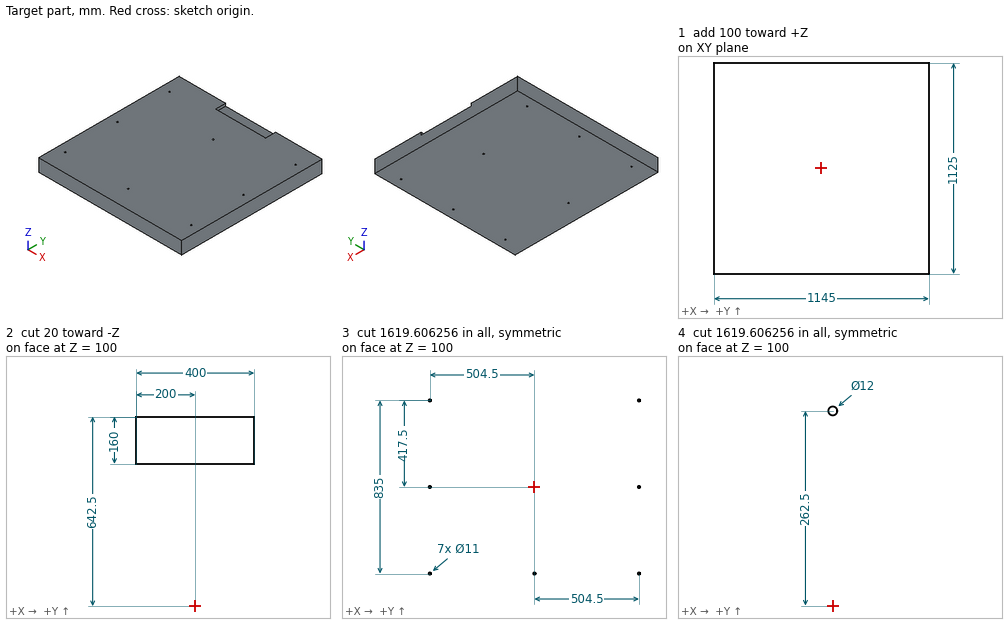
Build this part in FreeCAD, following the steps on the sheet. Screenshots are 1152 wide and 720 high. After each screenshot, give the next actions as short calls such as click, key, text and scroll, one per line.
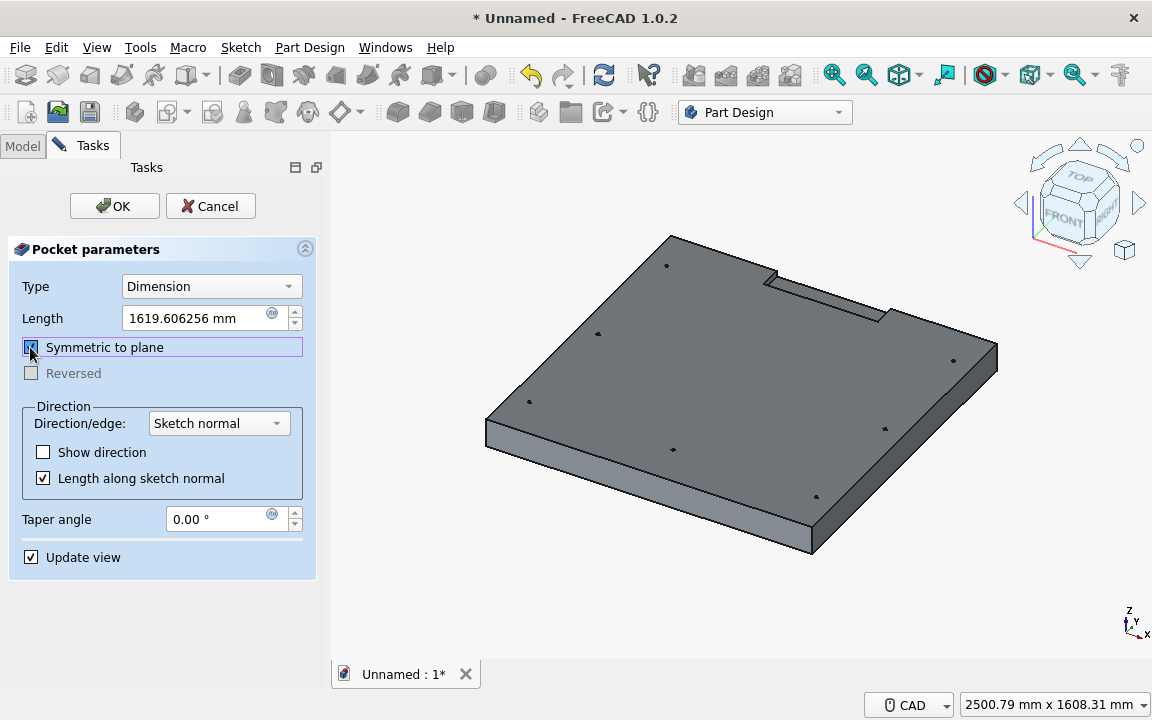
click(115, 206)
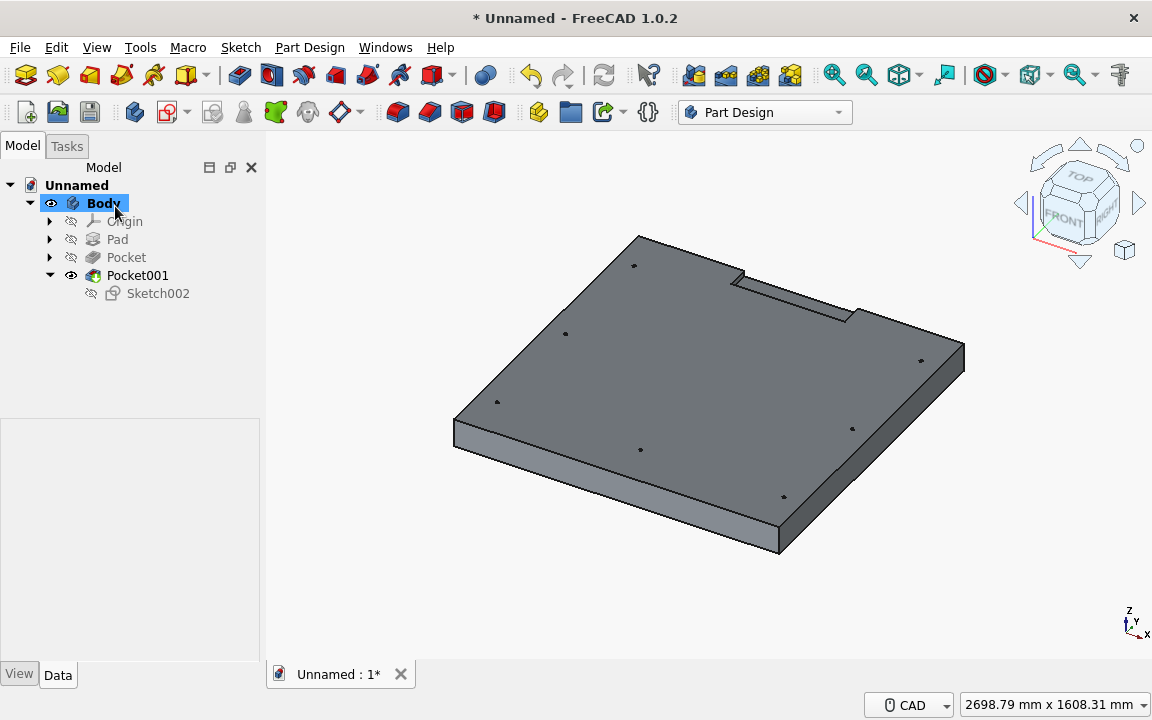
click(709, 381)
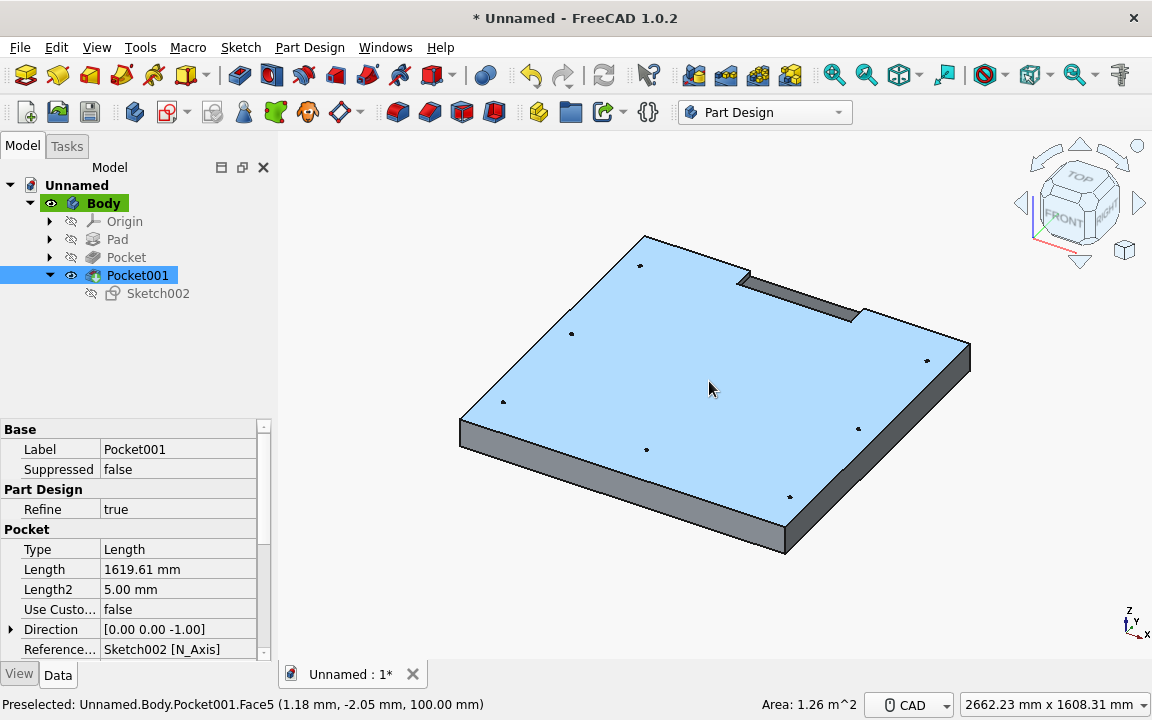
click(168, 112)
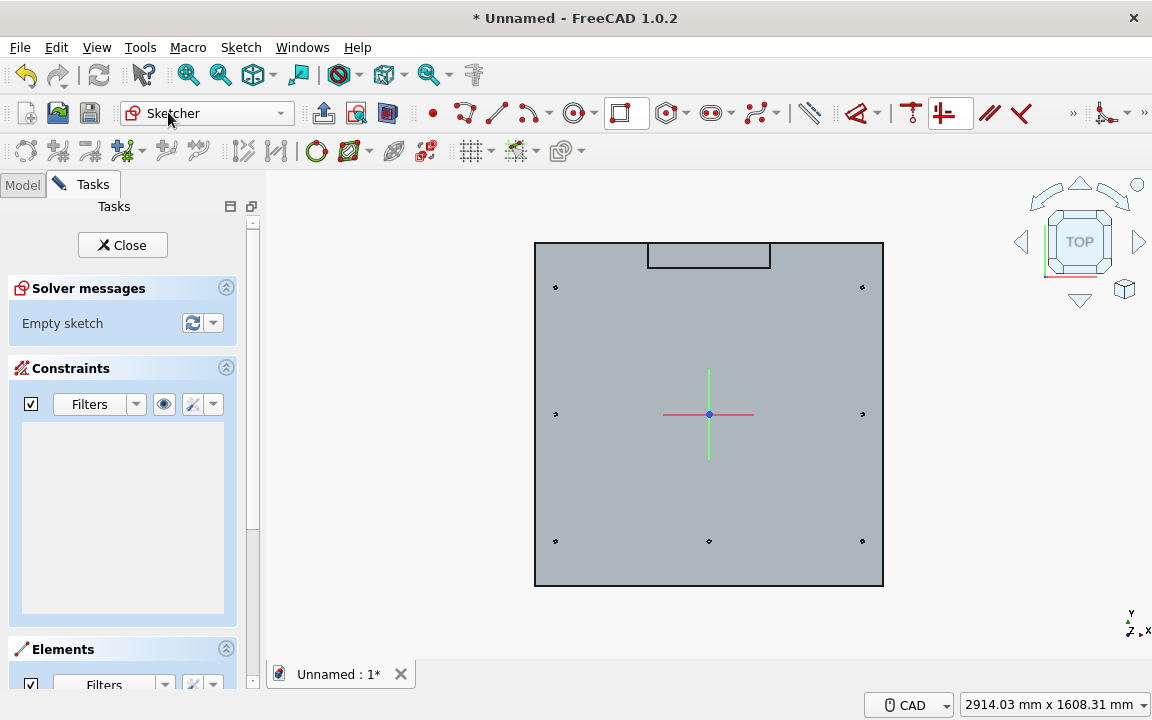
scroll(713, 331, up, 15)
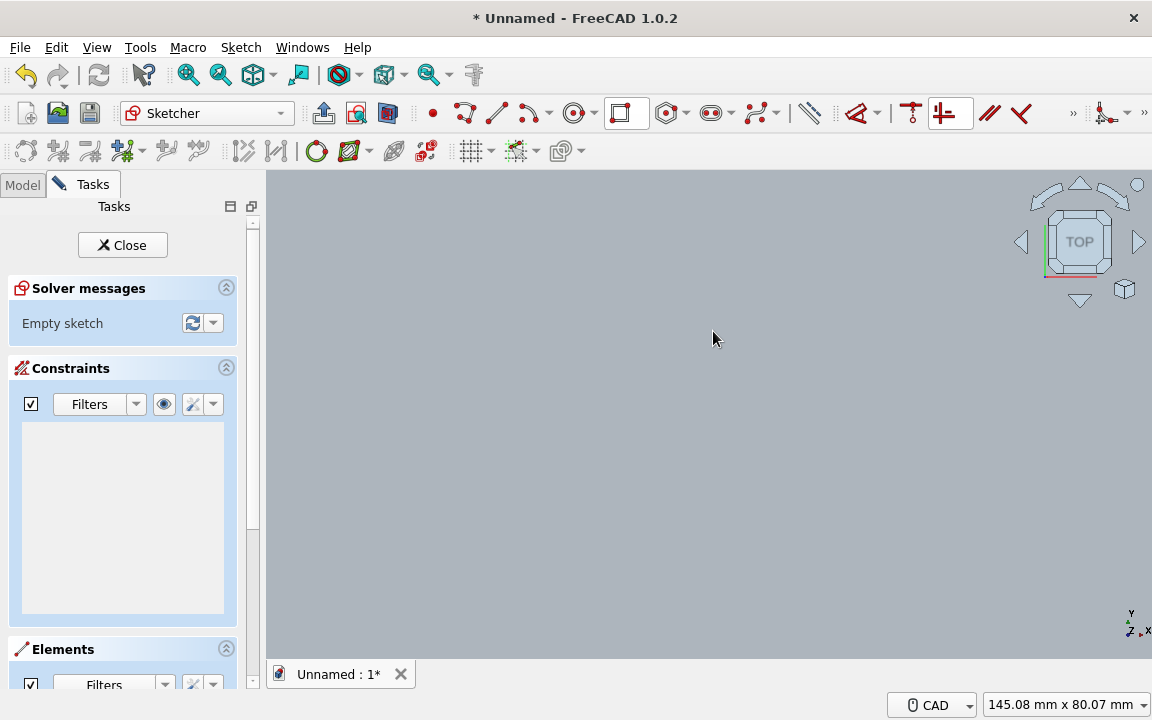
scroll(617, 394, up, 7)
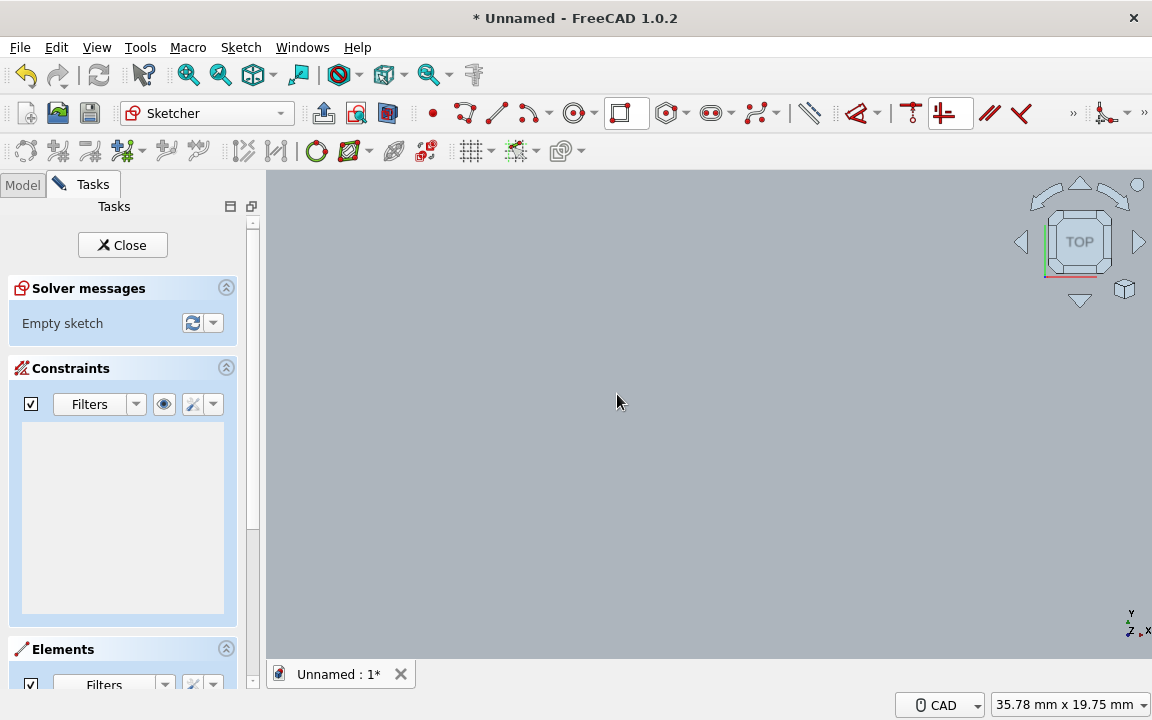
key(g)
key(c)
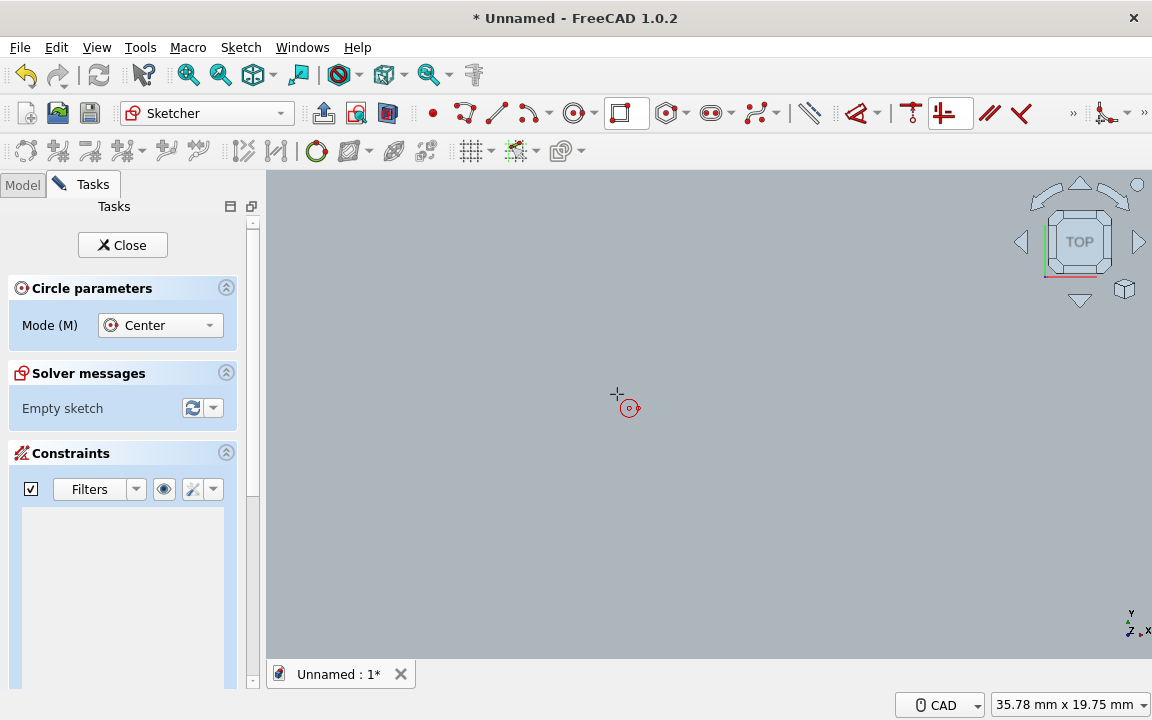
click(640, 412)
click(745, 307)
key(Escape)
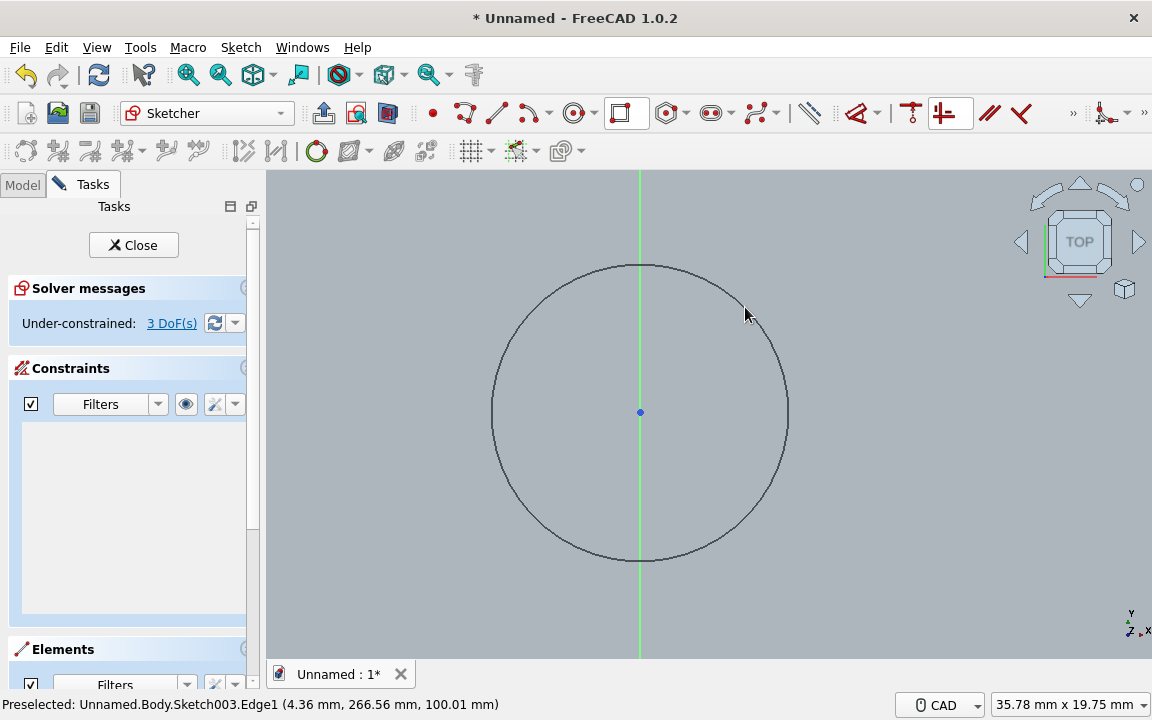
click(640, 413)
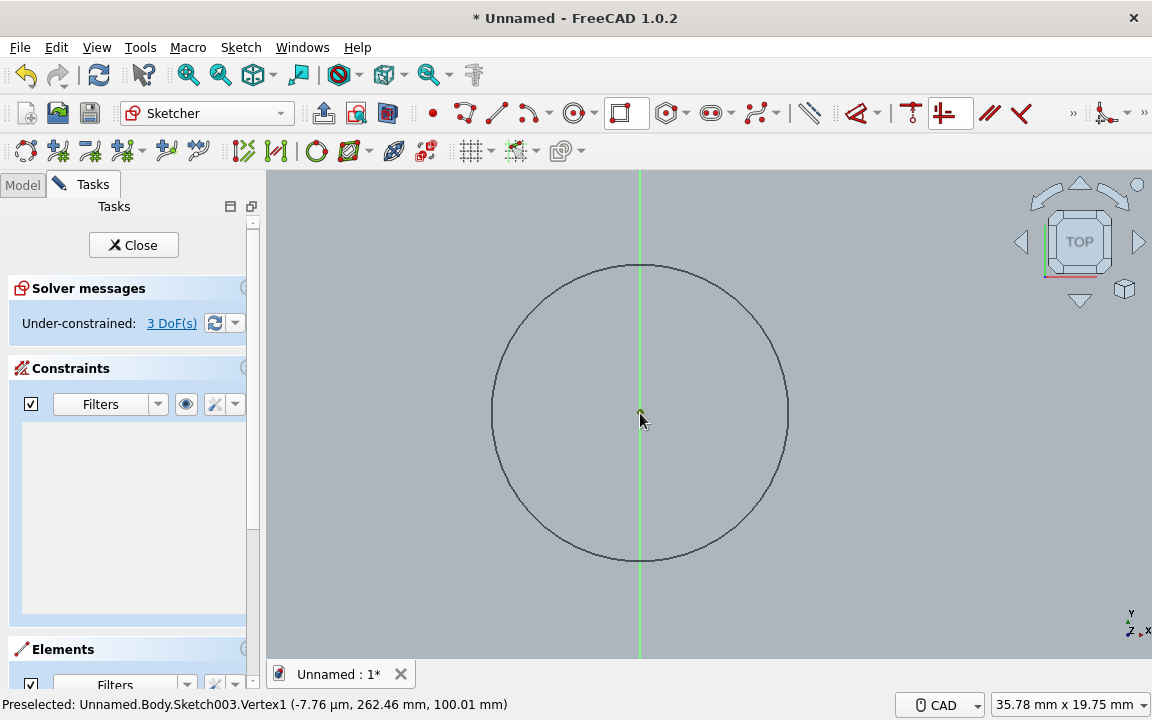
click(640, 600)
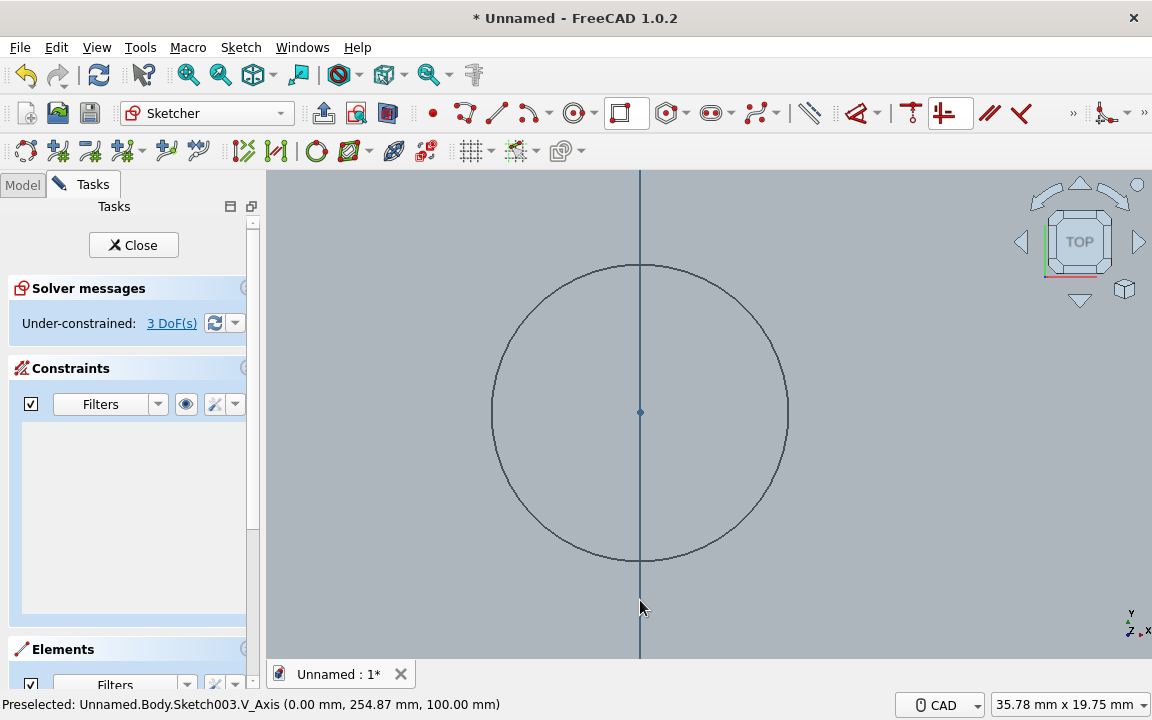
key(c)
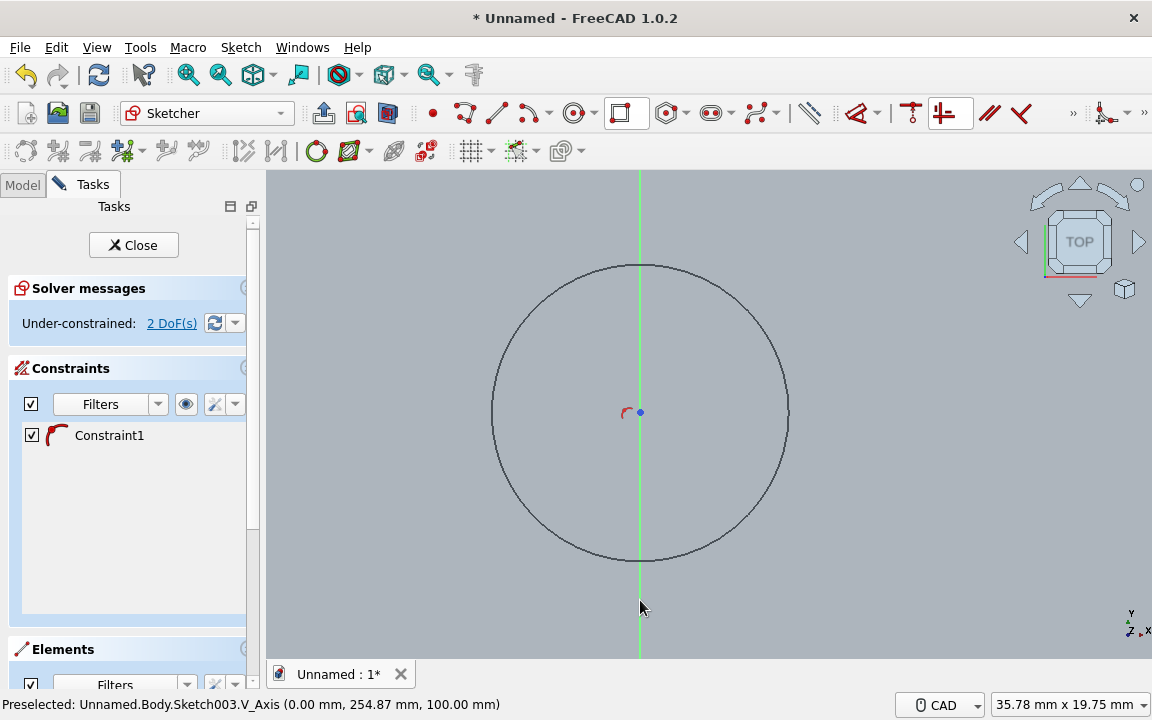
click(856, 114)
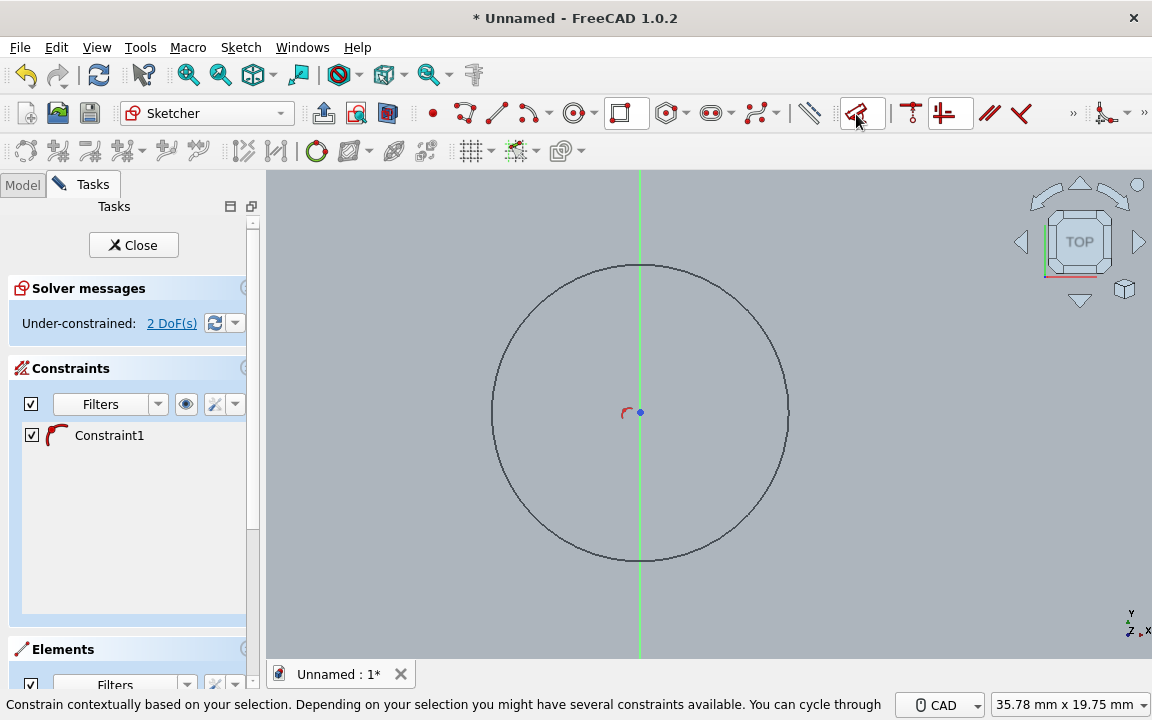
click(745, 308)
click(768, 285)